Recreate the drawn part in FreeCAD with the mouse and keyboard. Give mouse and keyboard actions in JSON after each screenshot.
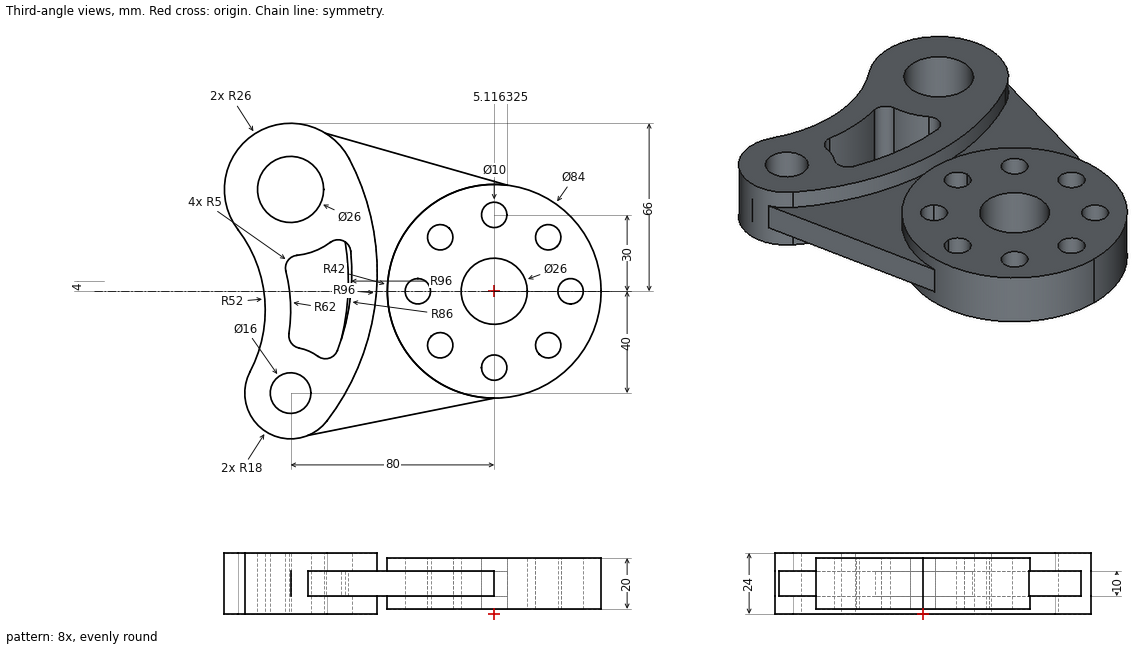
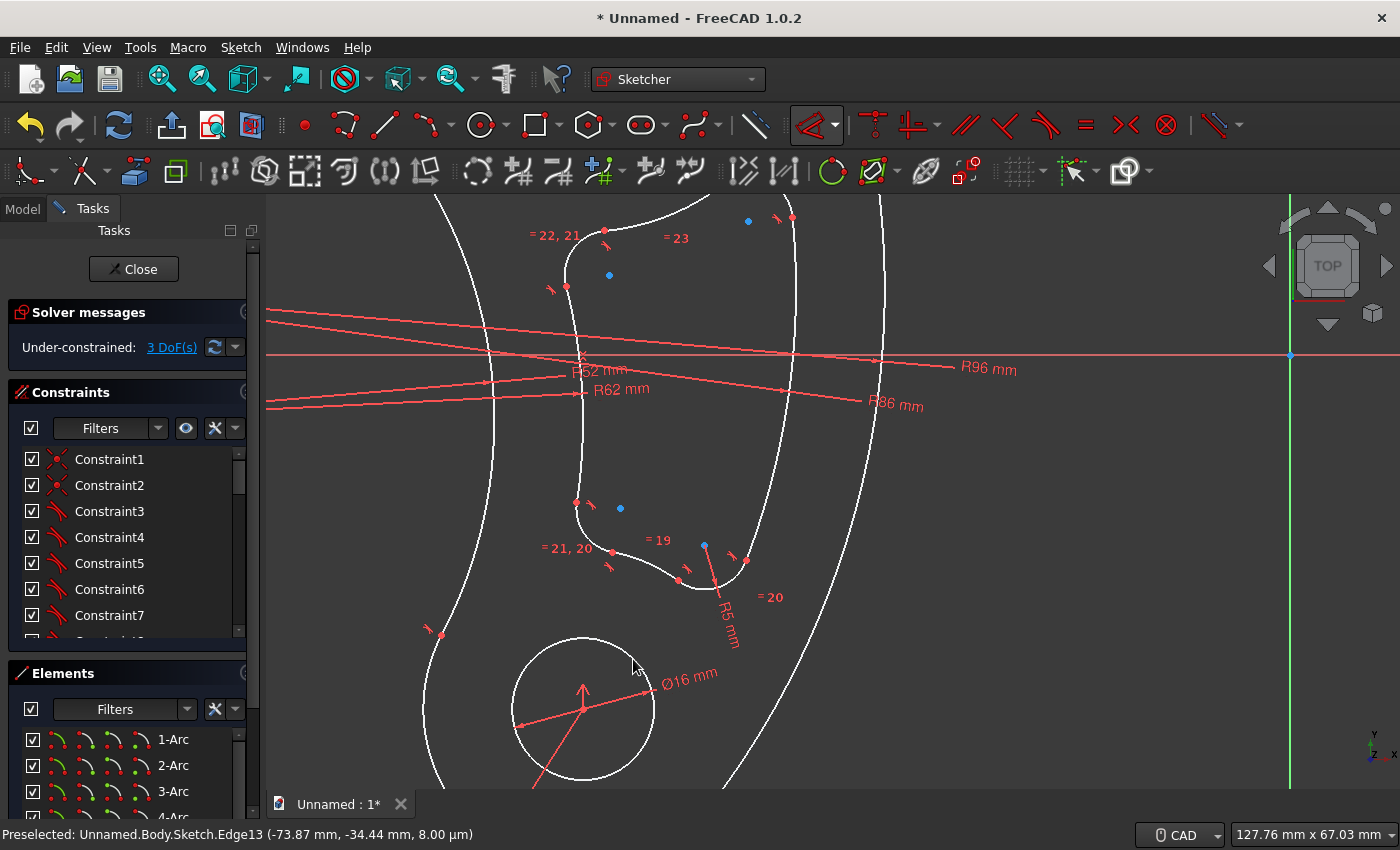
{"action": "scroll", "coordinate": [718, 588], "scroll_direction": "down", "scroll_amount": 5}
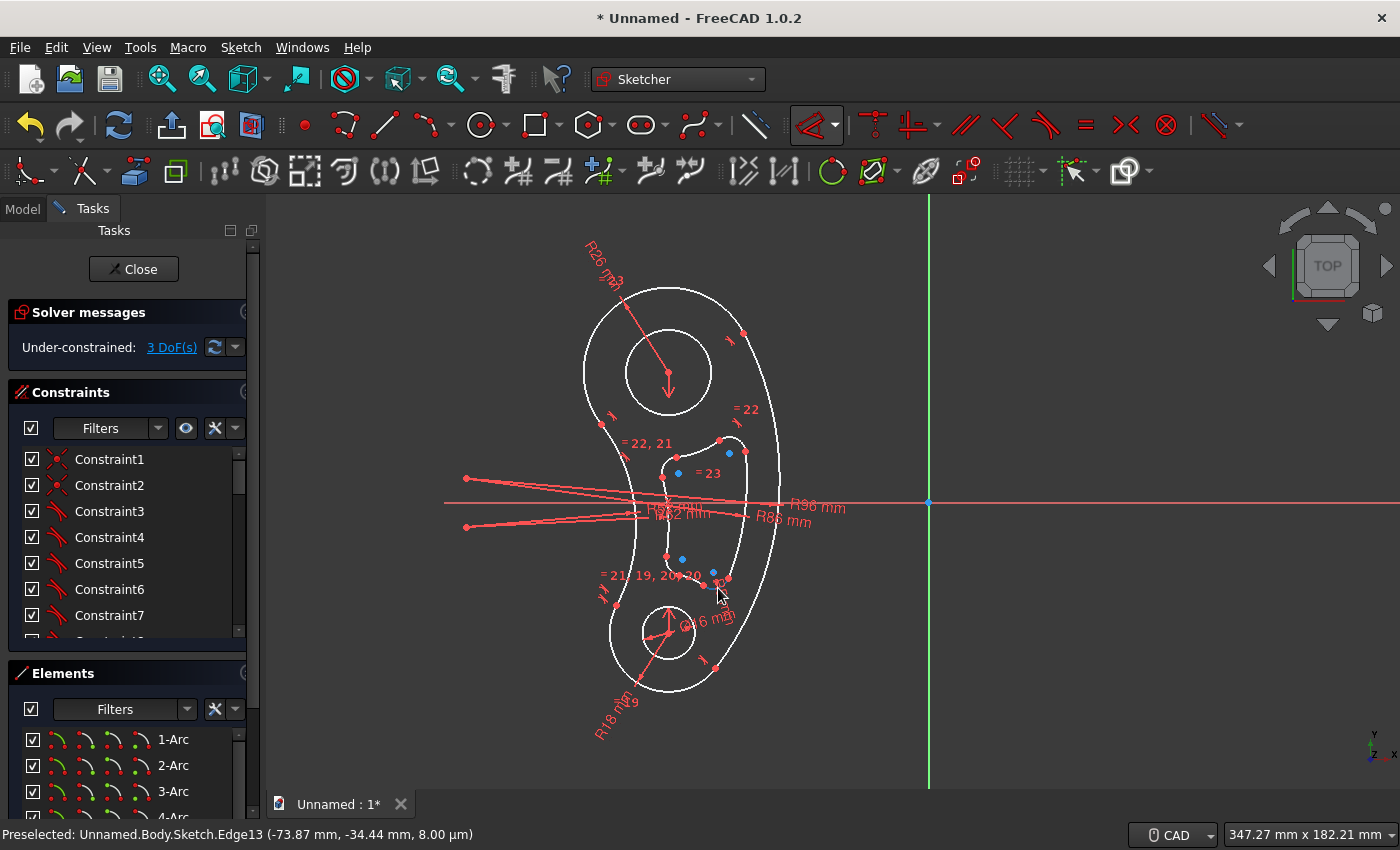
{"action": "left_click", "coordinate": [699, 342]}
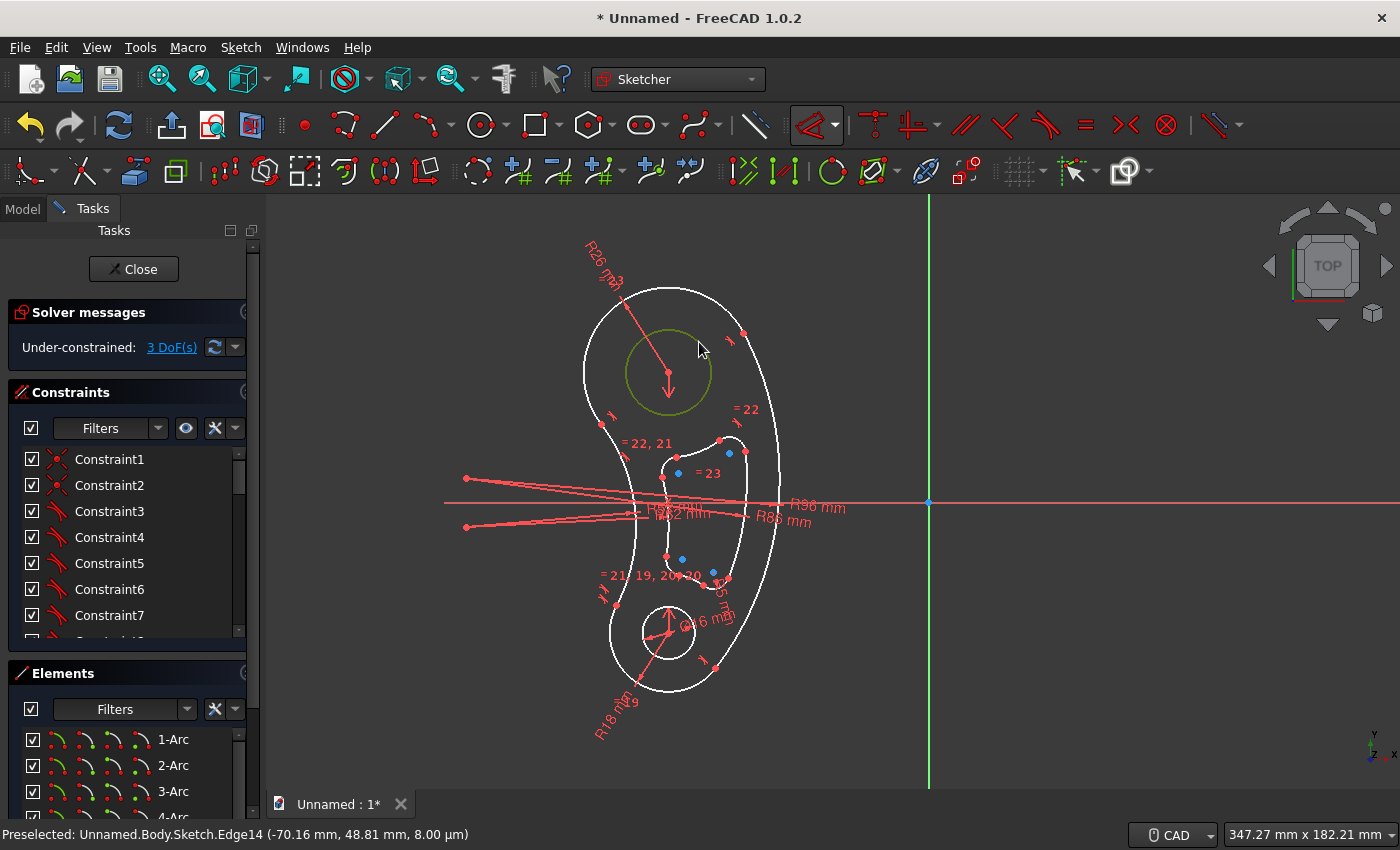
{"action": "key", "text": "k o"}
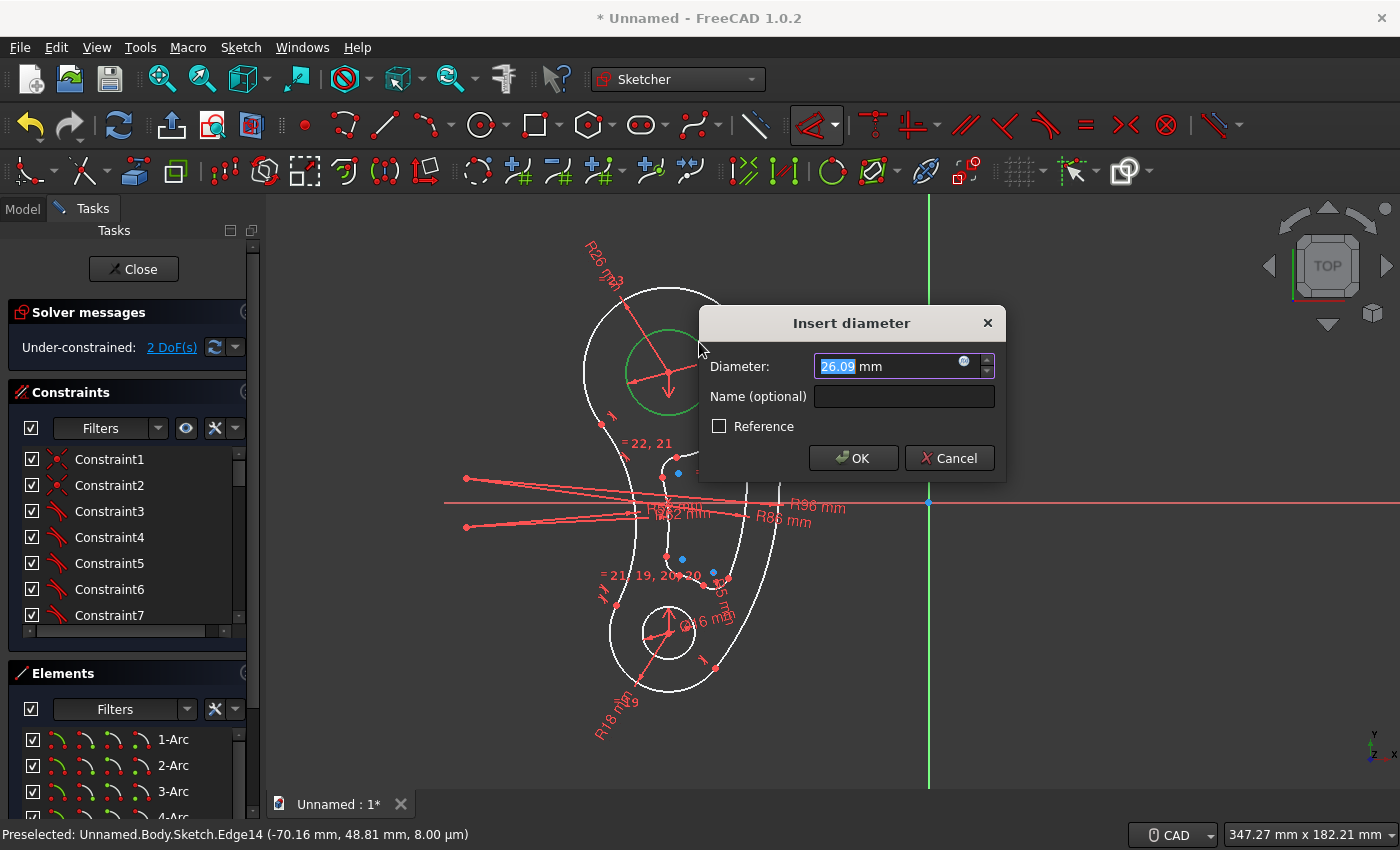
{"action": "type", "text": "26"}
{"action": "key", "text": "Return"}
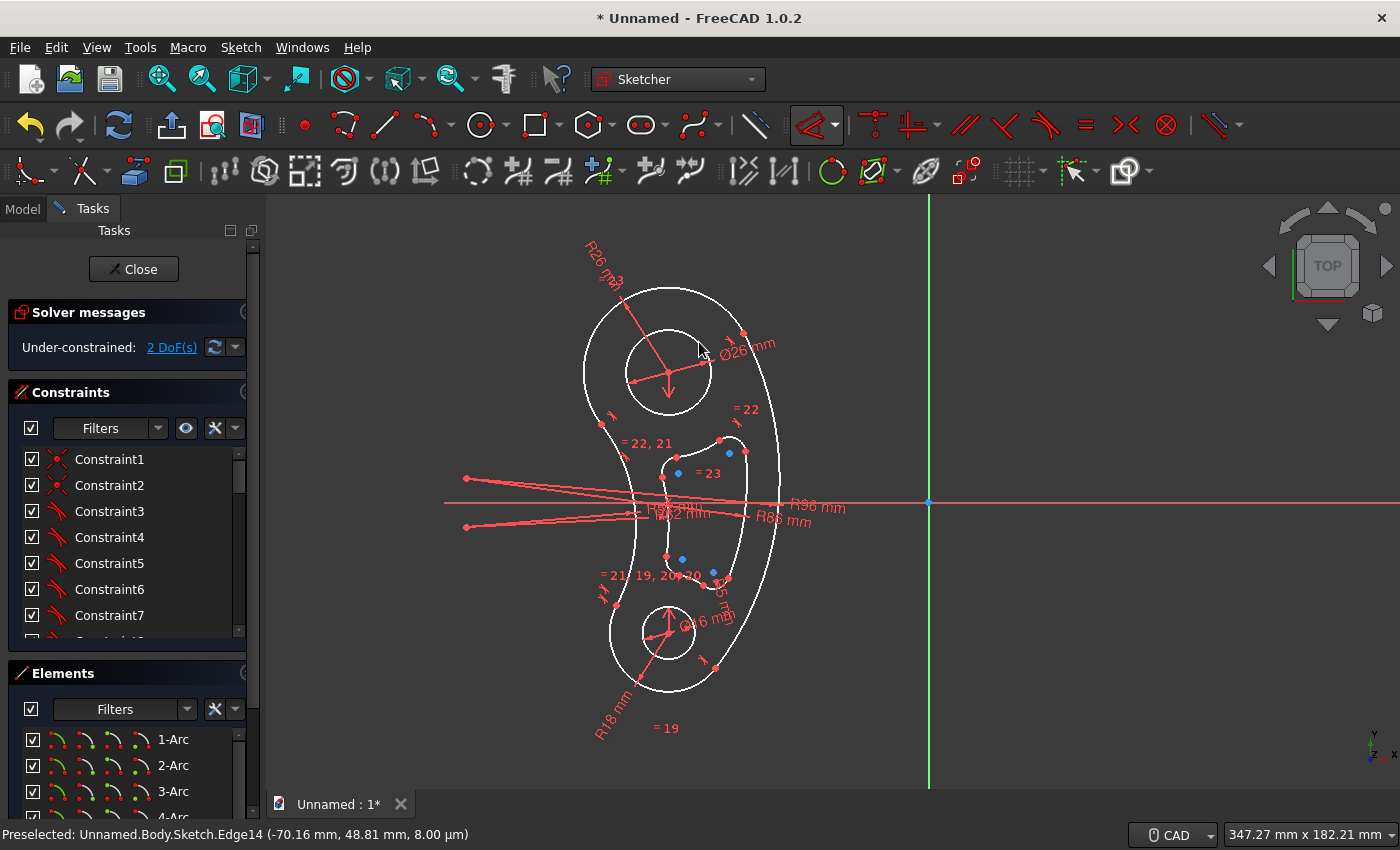
{"action": "left_click", "coordinate": [669, 633]}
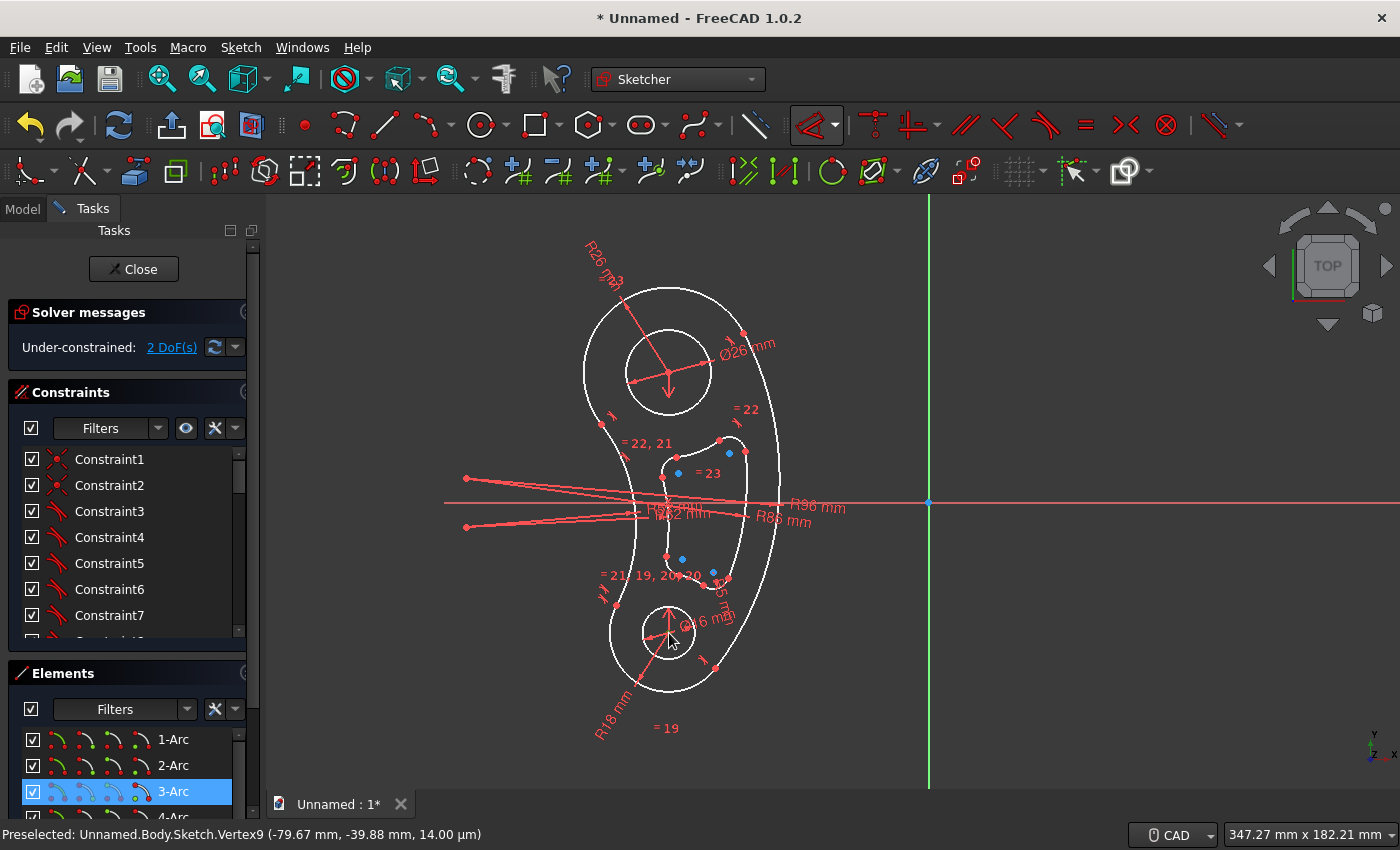
{"action": "left_click", "coordinate": [838, 126]}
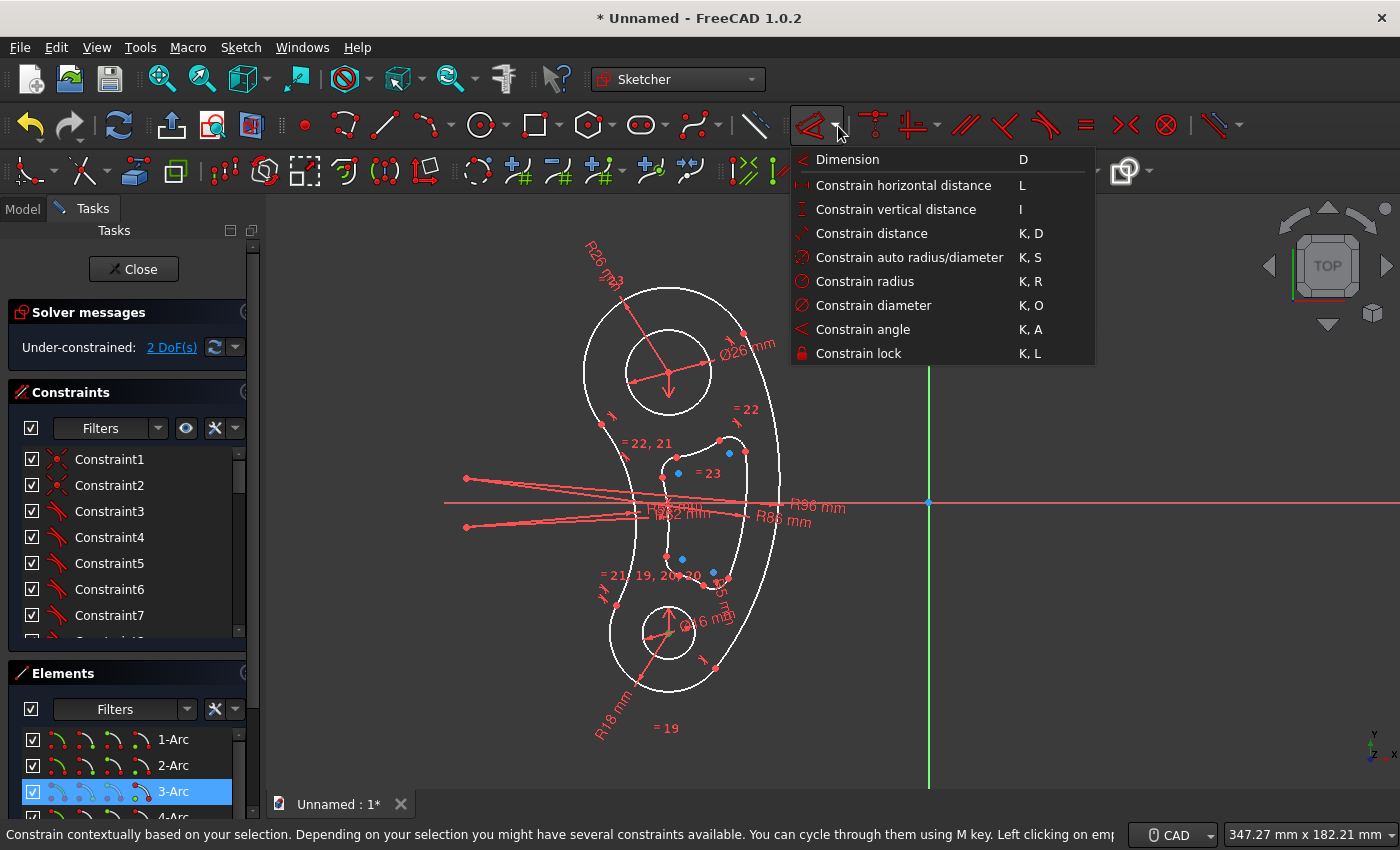
{"action": "left_click", "coordinate": [943, 185]}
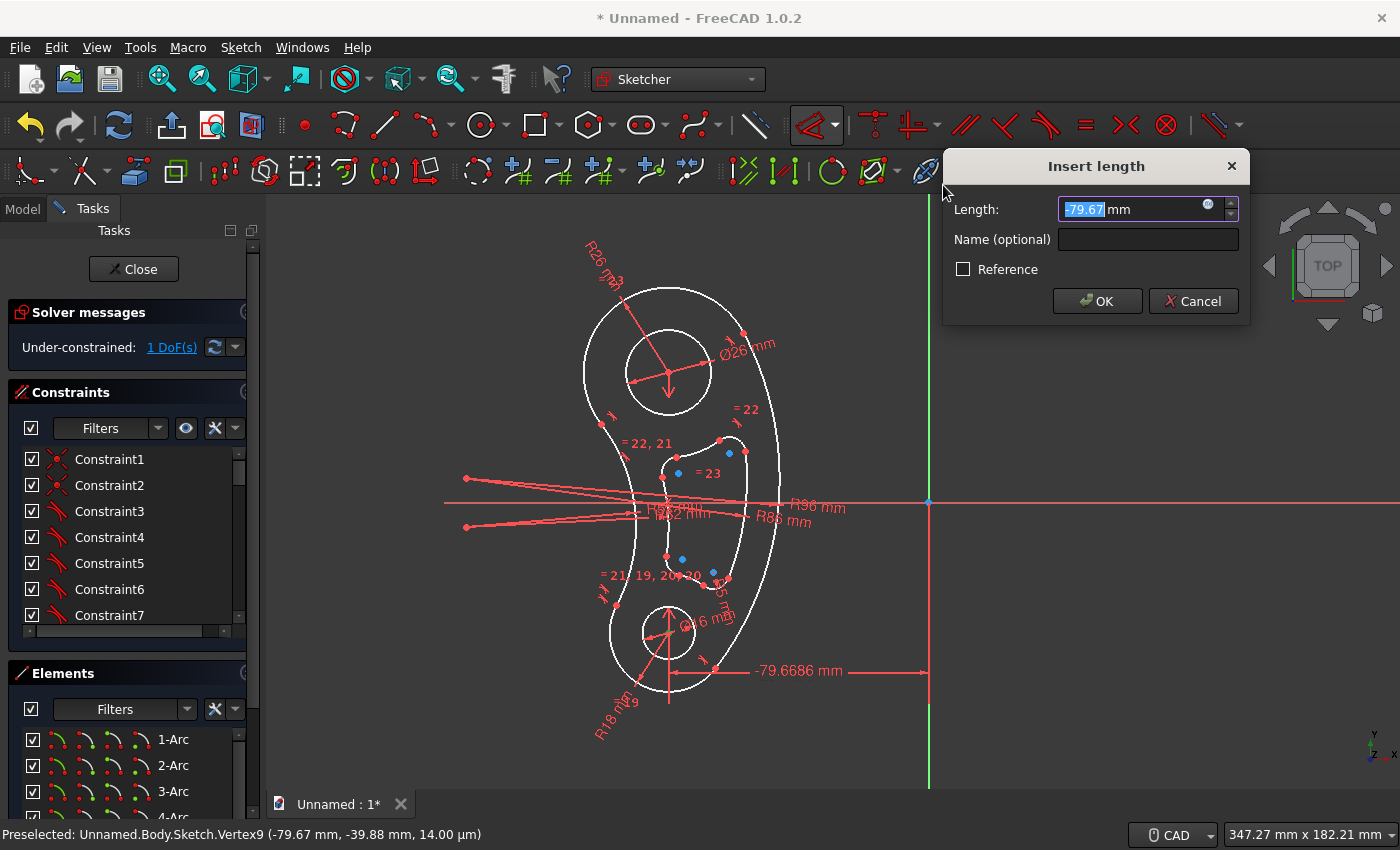
{"action": "type", "text": "-80"}
{"action": "key", "text": "Return"}